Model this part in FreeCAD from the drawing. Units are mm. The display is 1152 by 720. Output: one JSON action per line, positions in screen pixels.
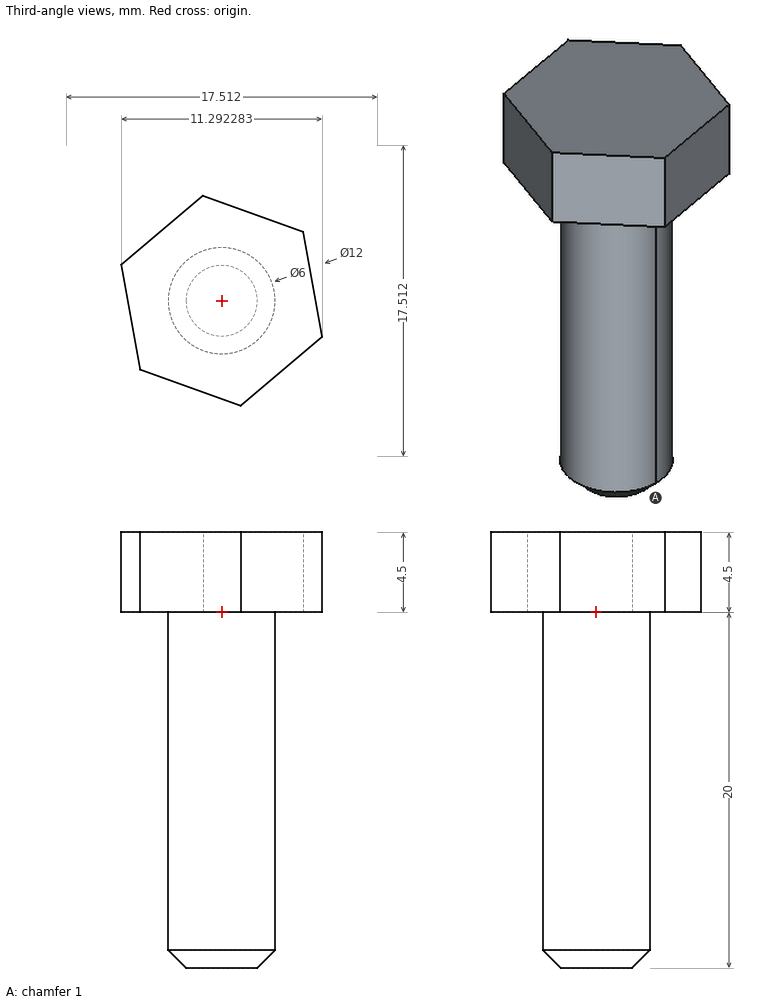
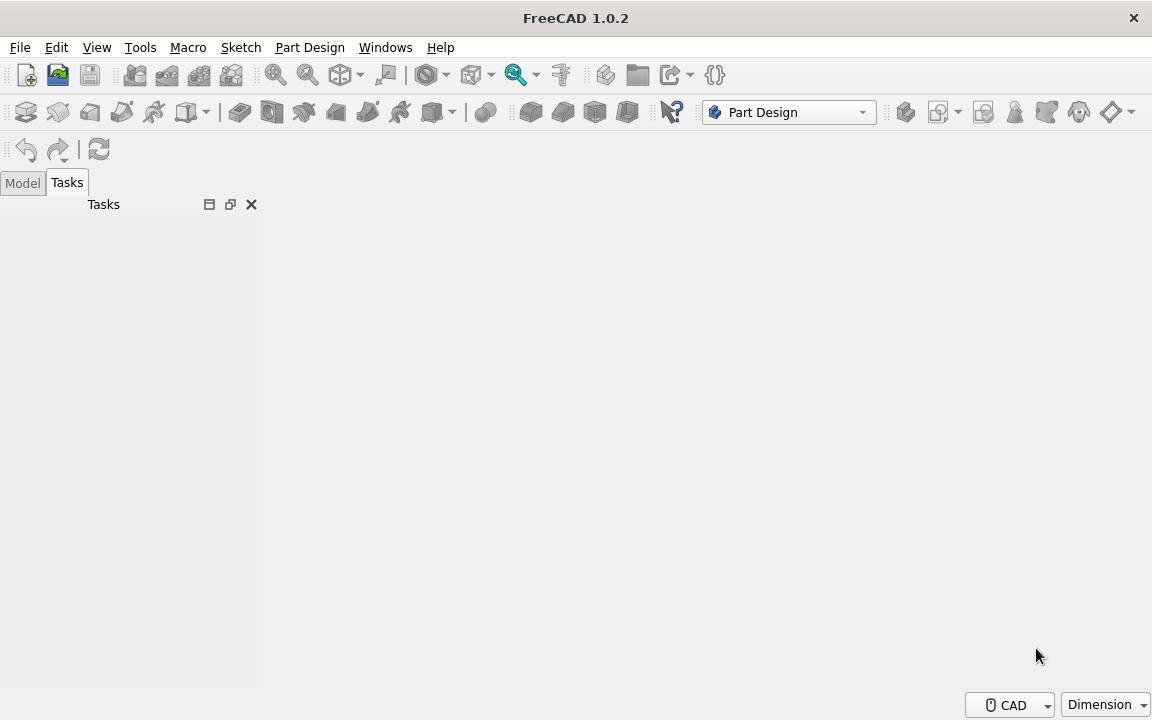
{"action": "key", "text": "ctrl+n"}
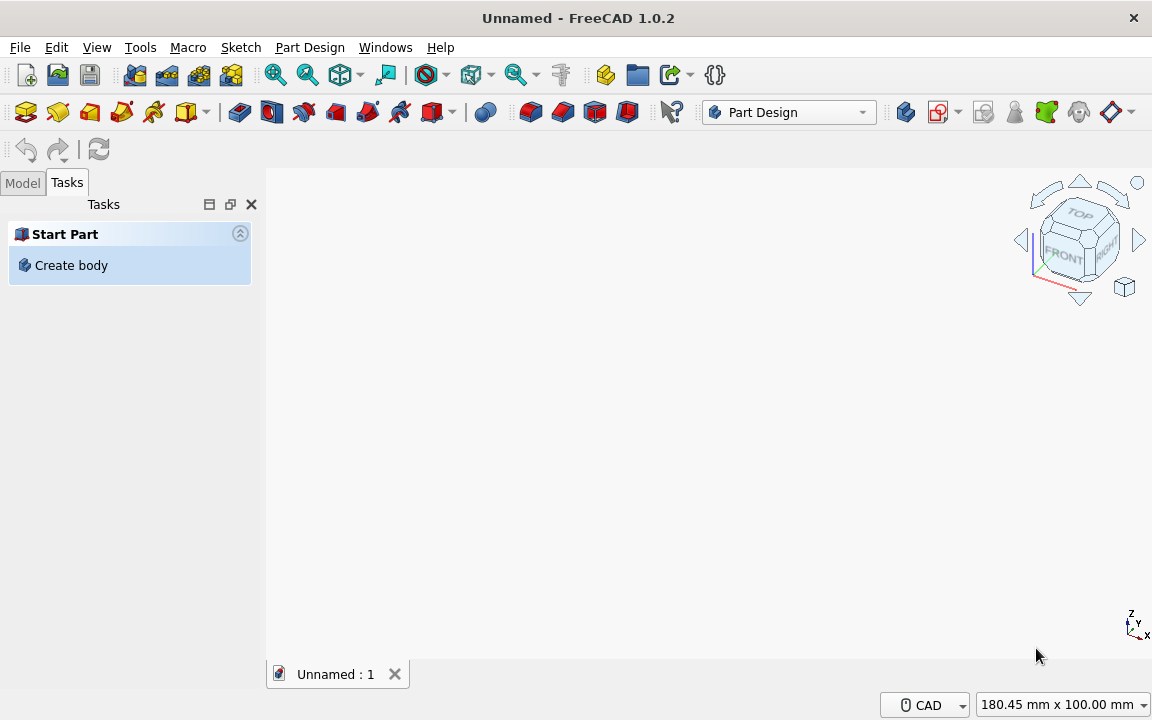
{"action": "left_click", "coordinate": [938, 112]}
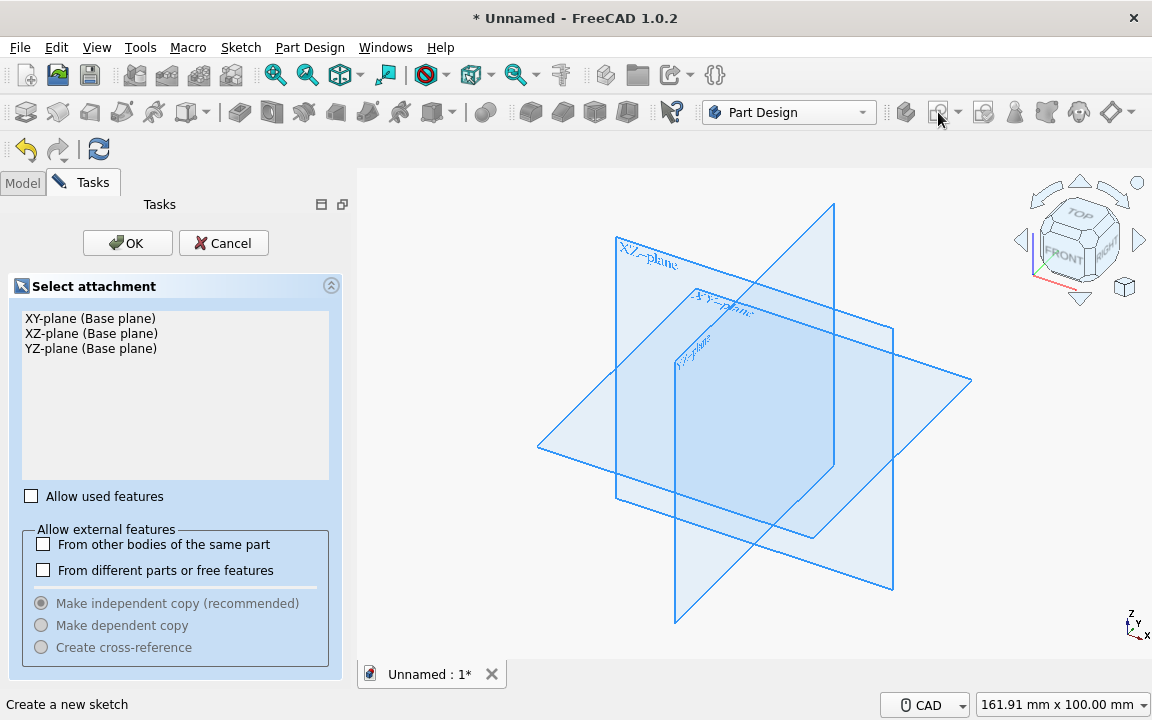
{"action": "left_click", "coordinate": [82, 318]}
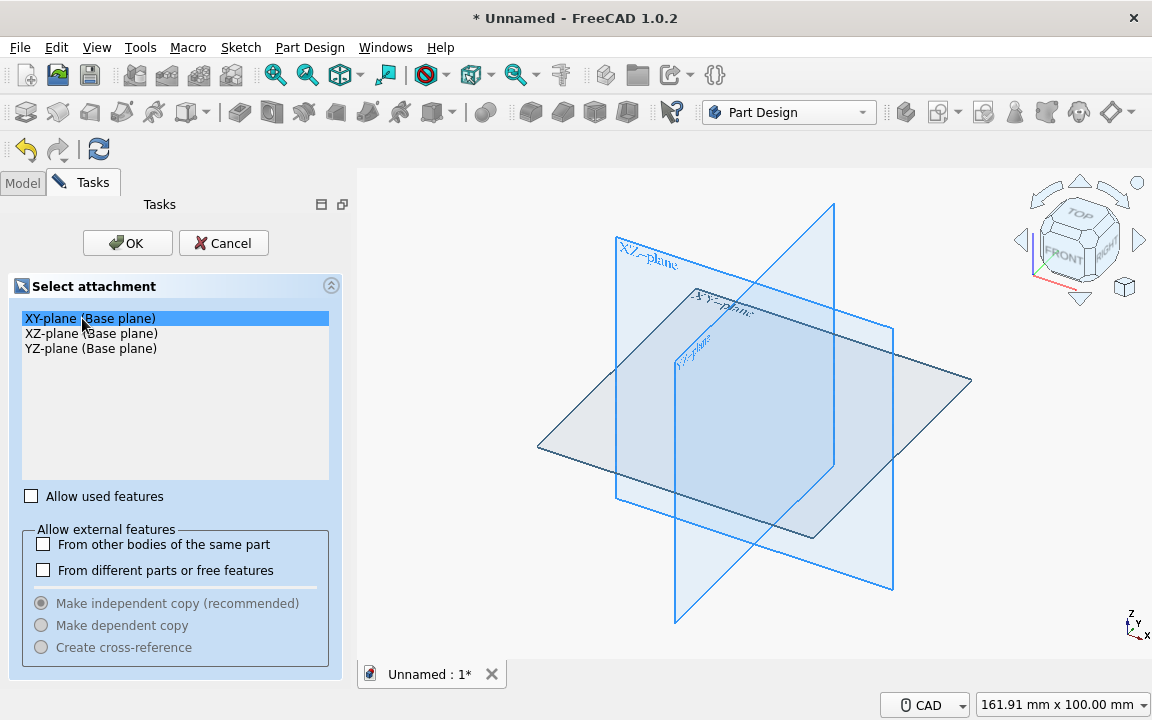
{"action": "left_click", "coordinate": [128, 243]}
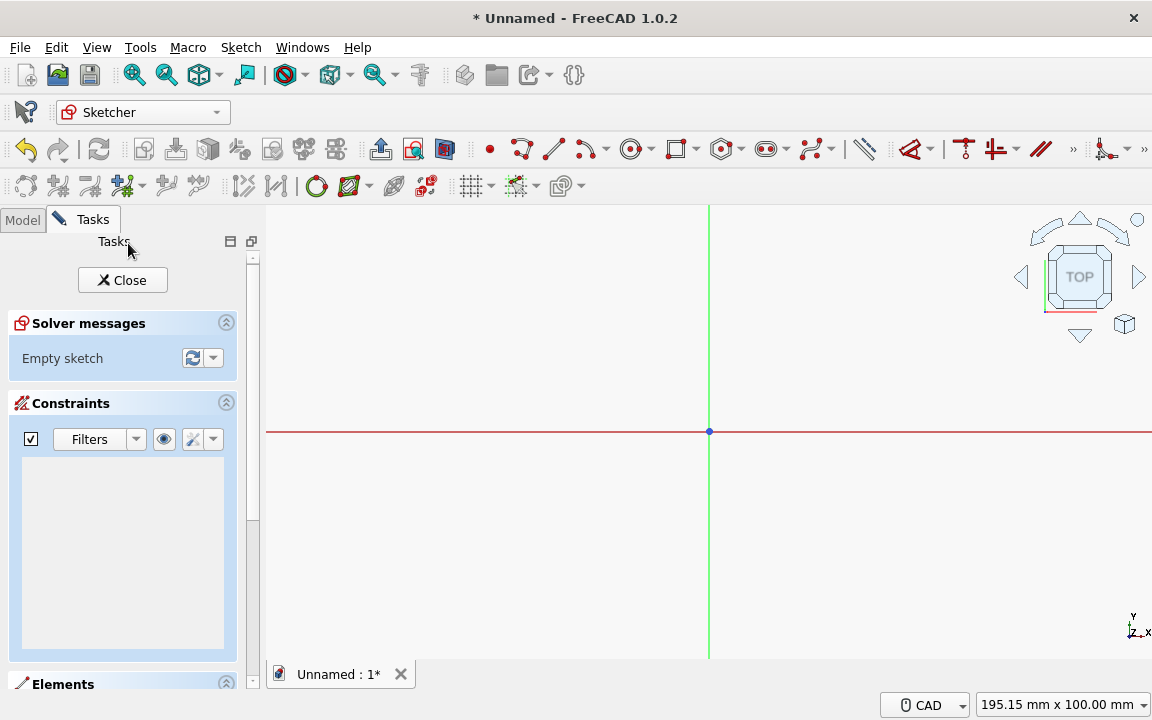
{"action": "scroll", "coordinate": [726, 432], "scroll_direction": "up", "scroll_amount": 8}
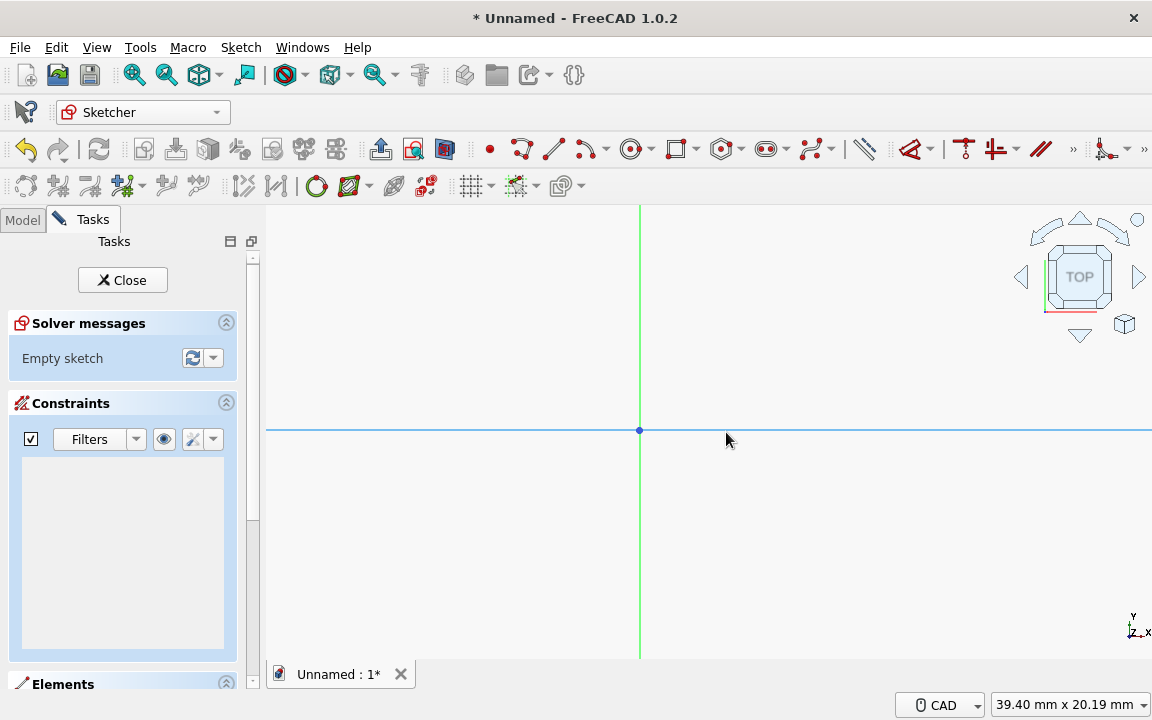
{"action": "key", "text": "g c"}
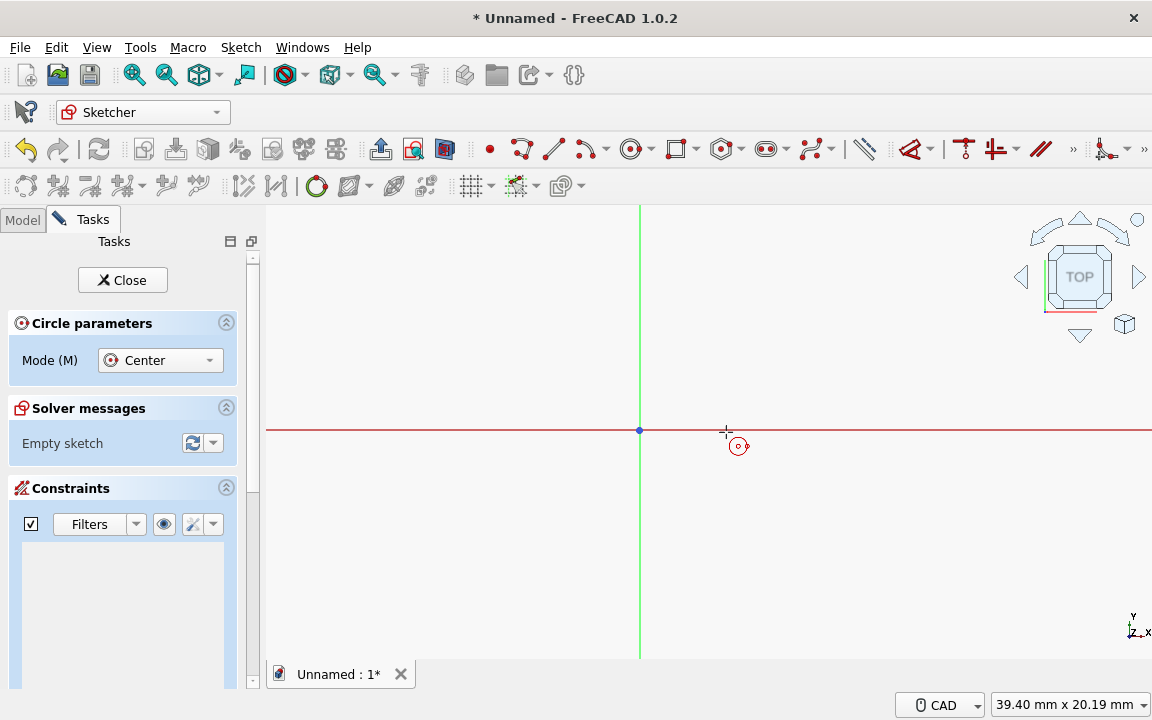
{"action": "left_click", "coordinate": [640, 430]}
{"action": "left_click", "coordinate": [735, 335]}
{"action": "key", "text": "Escape"}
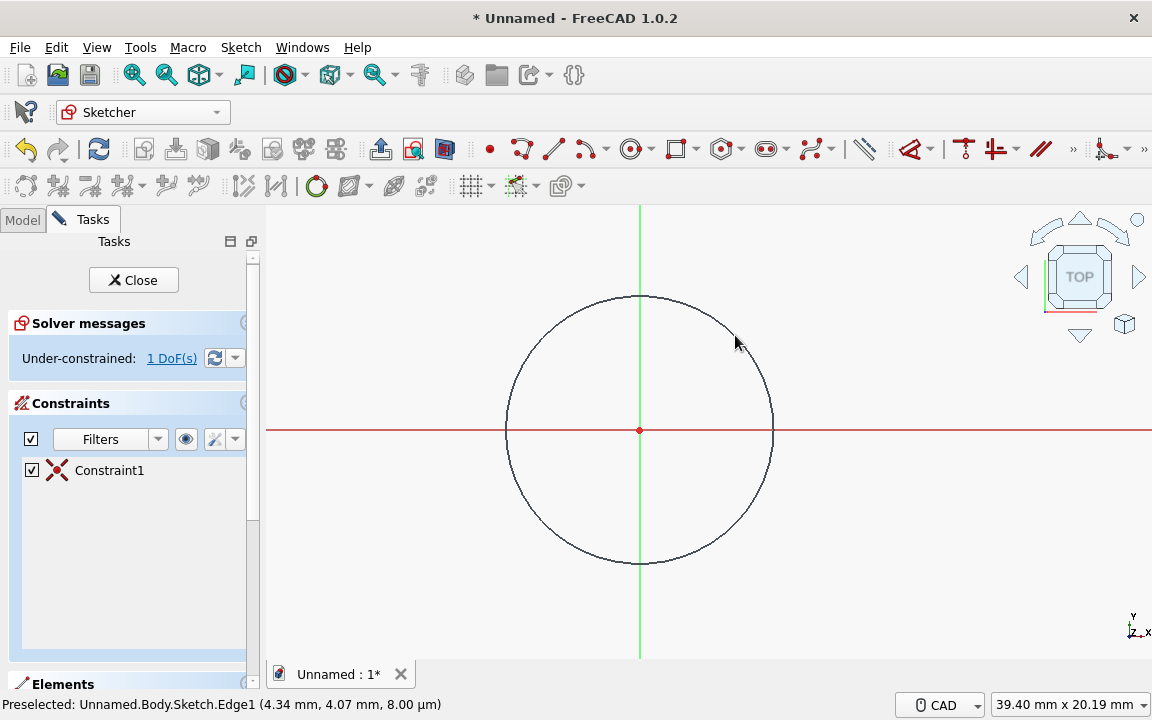
{"action": "key", "text": "d"}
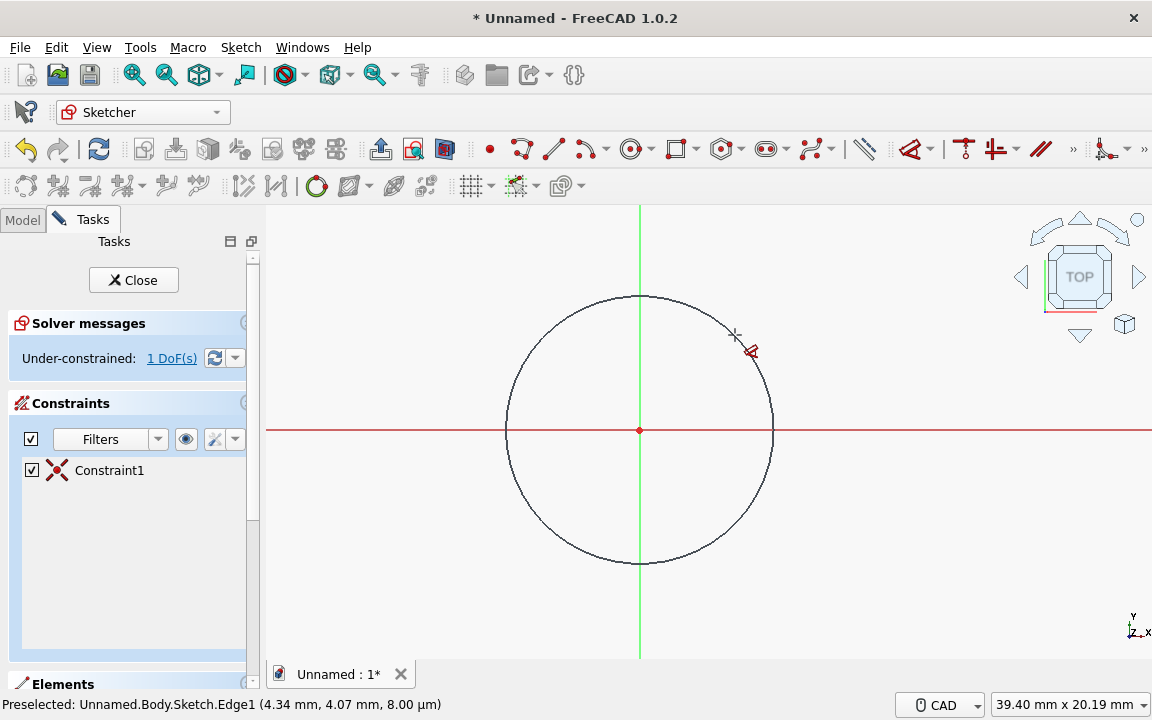
{"action": "left_click", "coordinate": [734, 335]}
{"action": "left_click", "coordinate": [757, 312]}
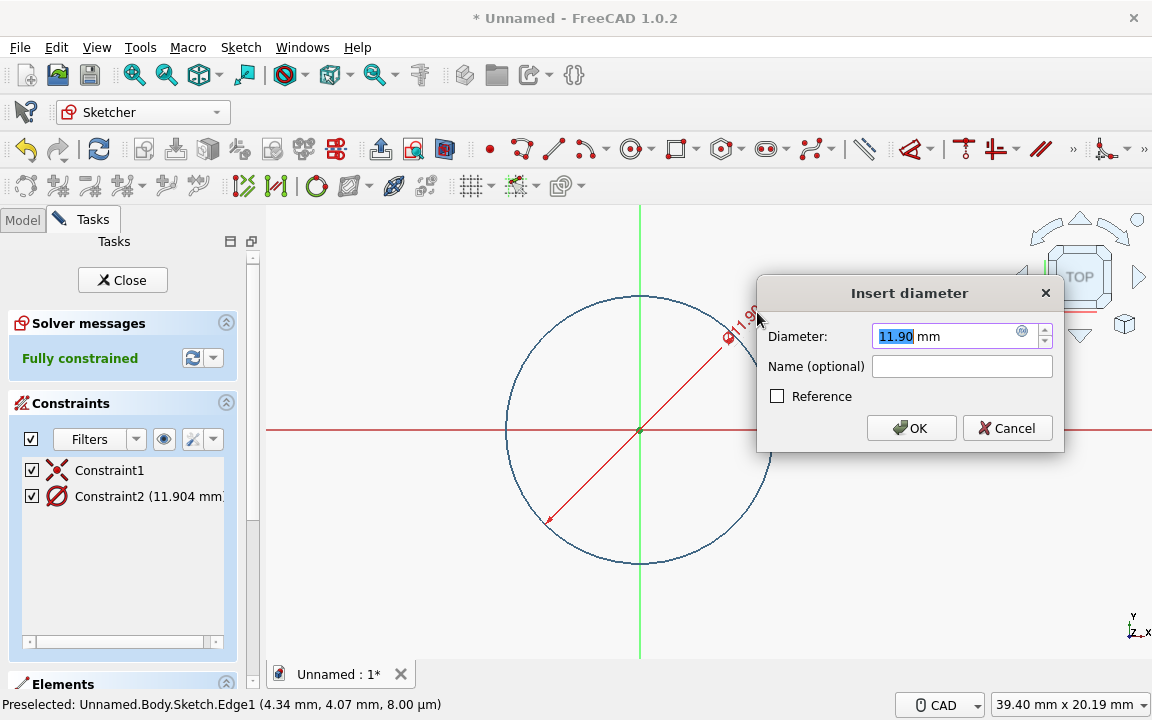
{"action": "type", "text": "12"}
{"action": "key", "text": "Return"}
{"action": "key", "text": "Escape"}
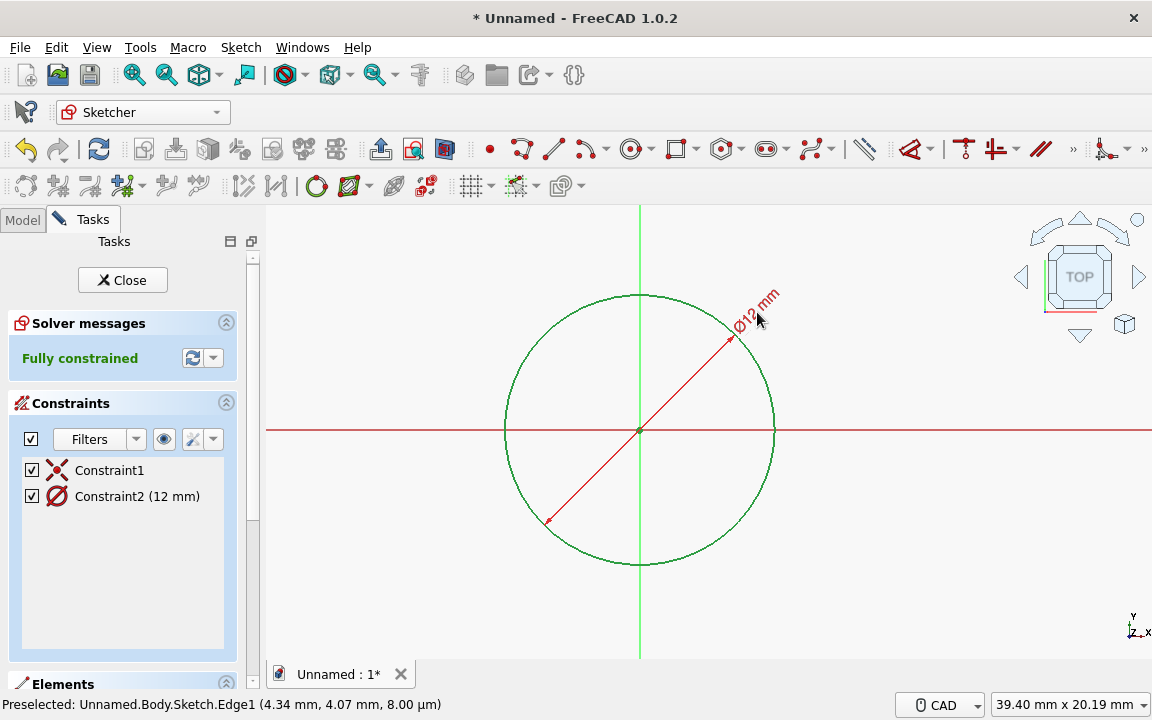
{"action": "left_click", "coordinate": [123, 280]}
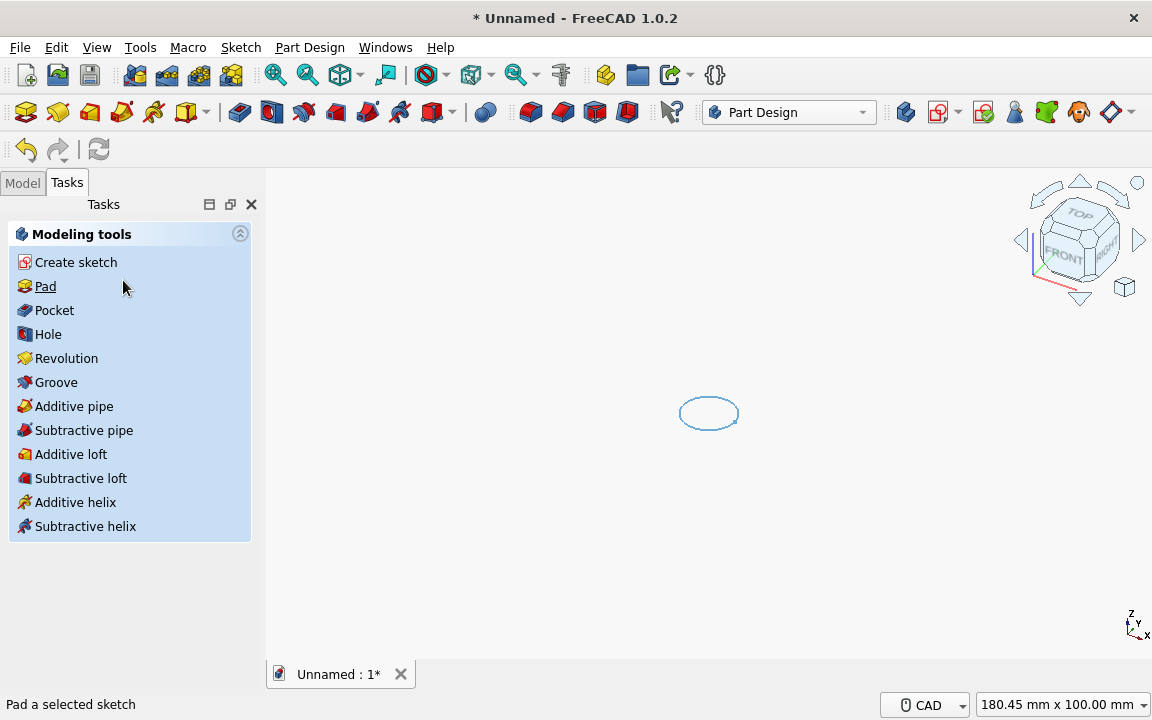
{"action": "left_click", "coordinate": [26, 112]}